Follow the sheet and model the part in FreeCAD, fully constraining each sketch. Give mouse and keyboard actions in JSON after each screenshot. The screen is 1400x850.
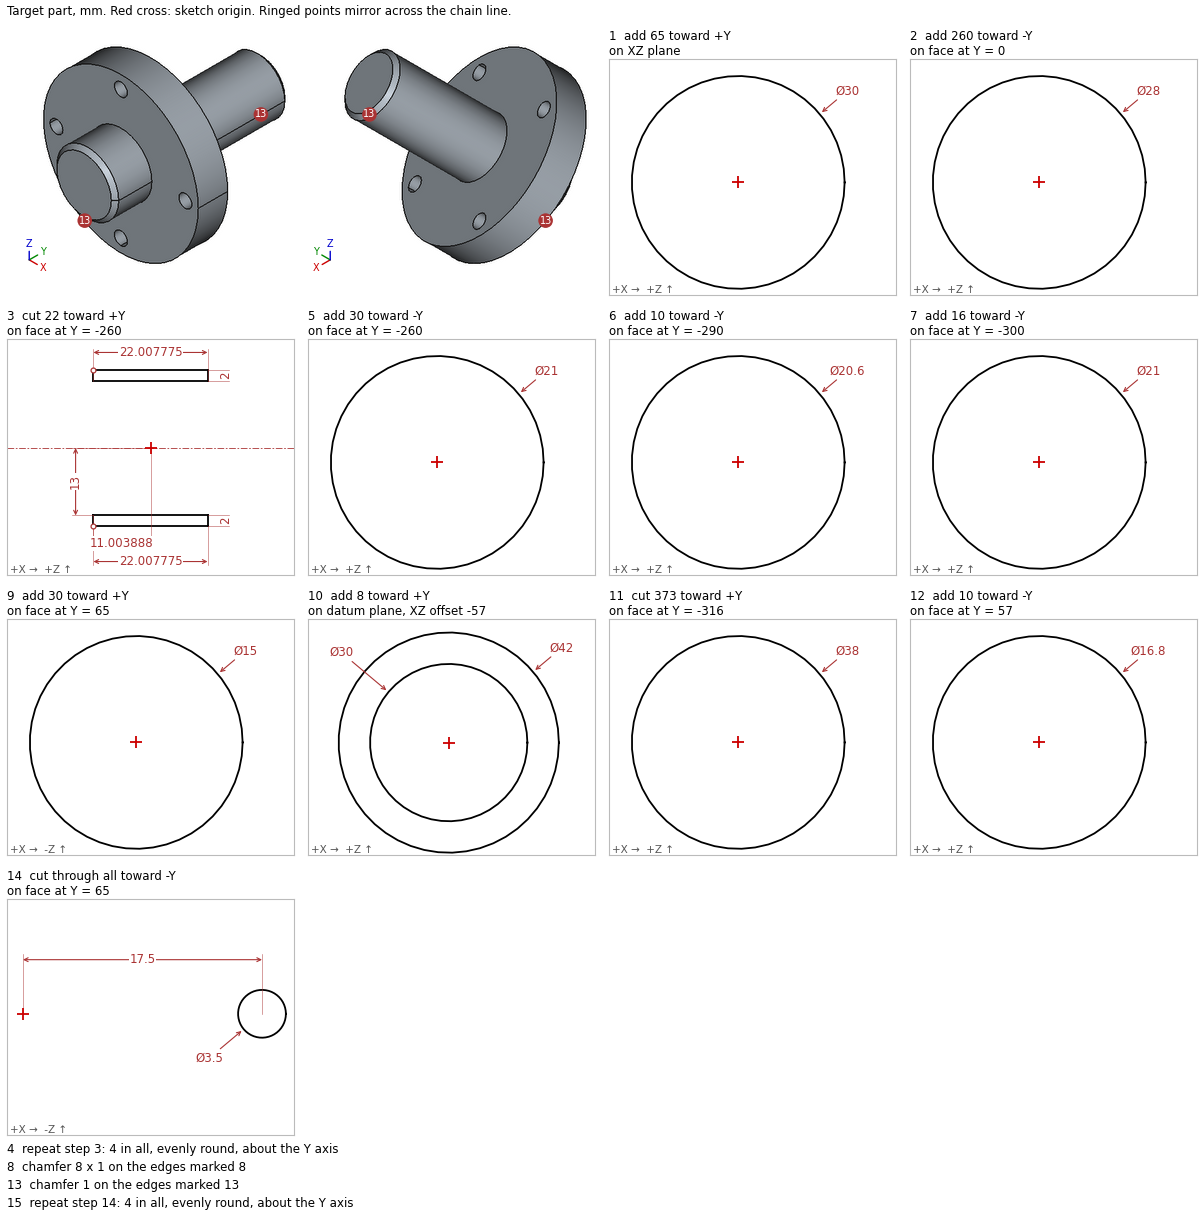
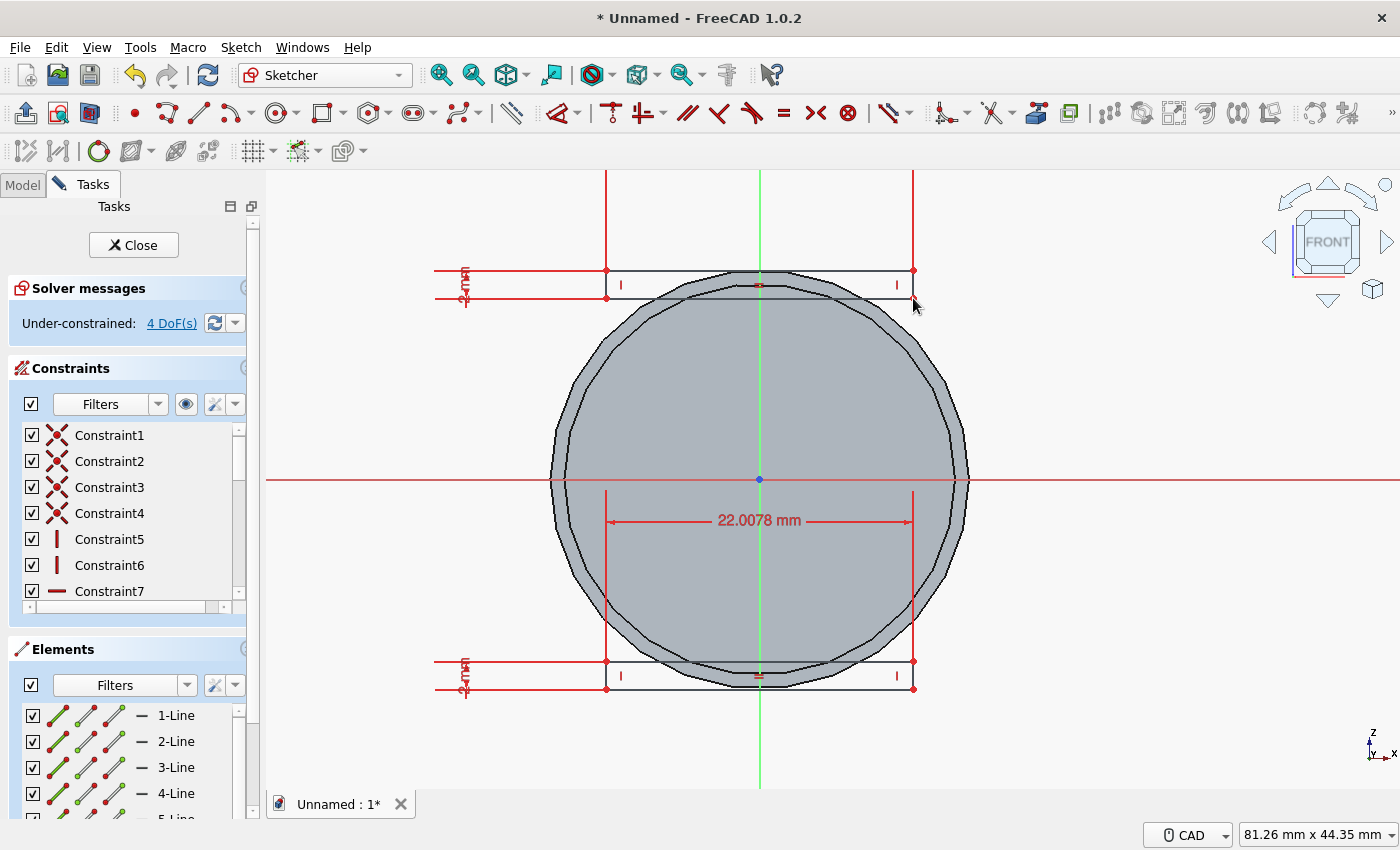
{"action": "left_click", "coordinate": [606, 690]}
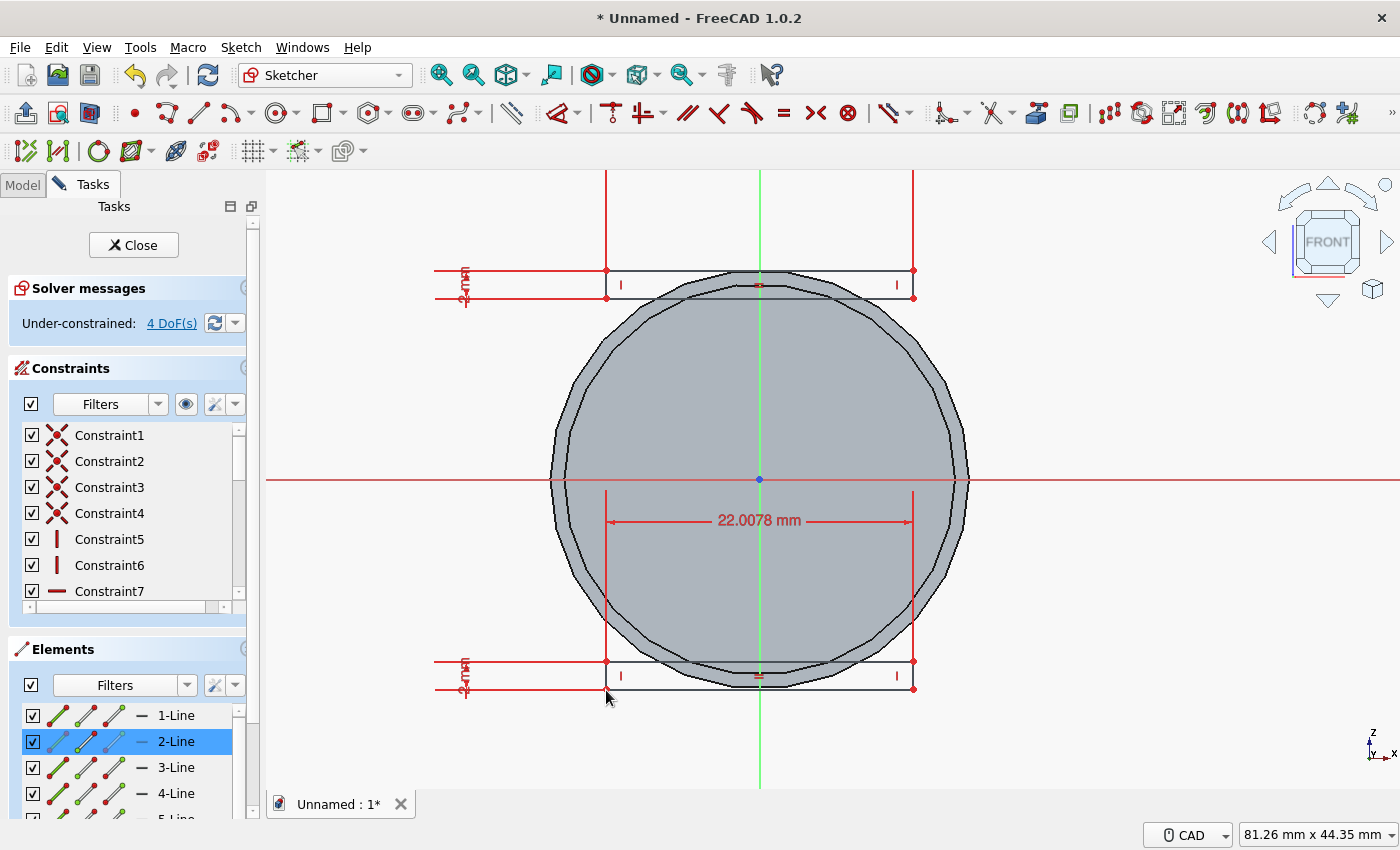
{"action": "left_click", "coordinate": [606, 271]}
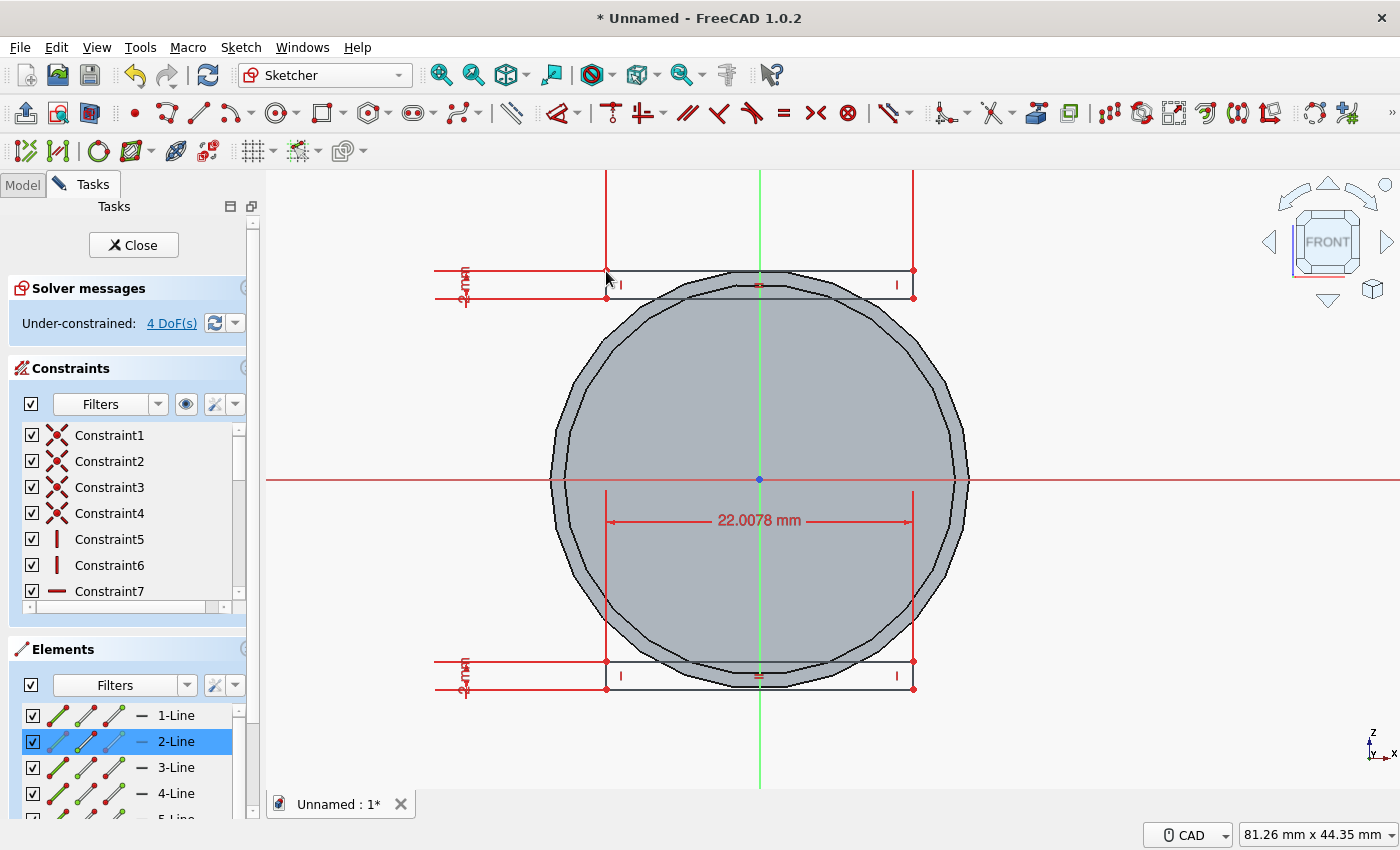
{"action": "left_click", "coordinate": [361, 480]}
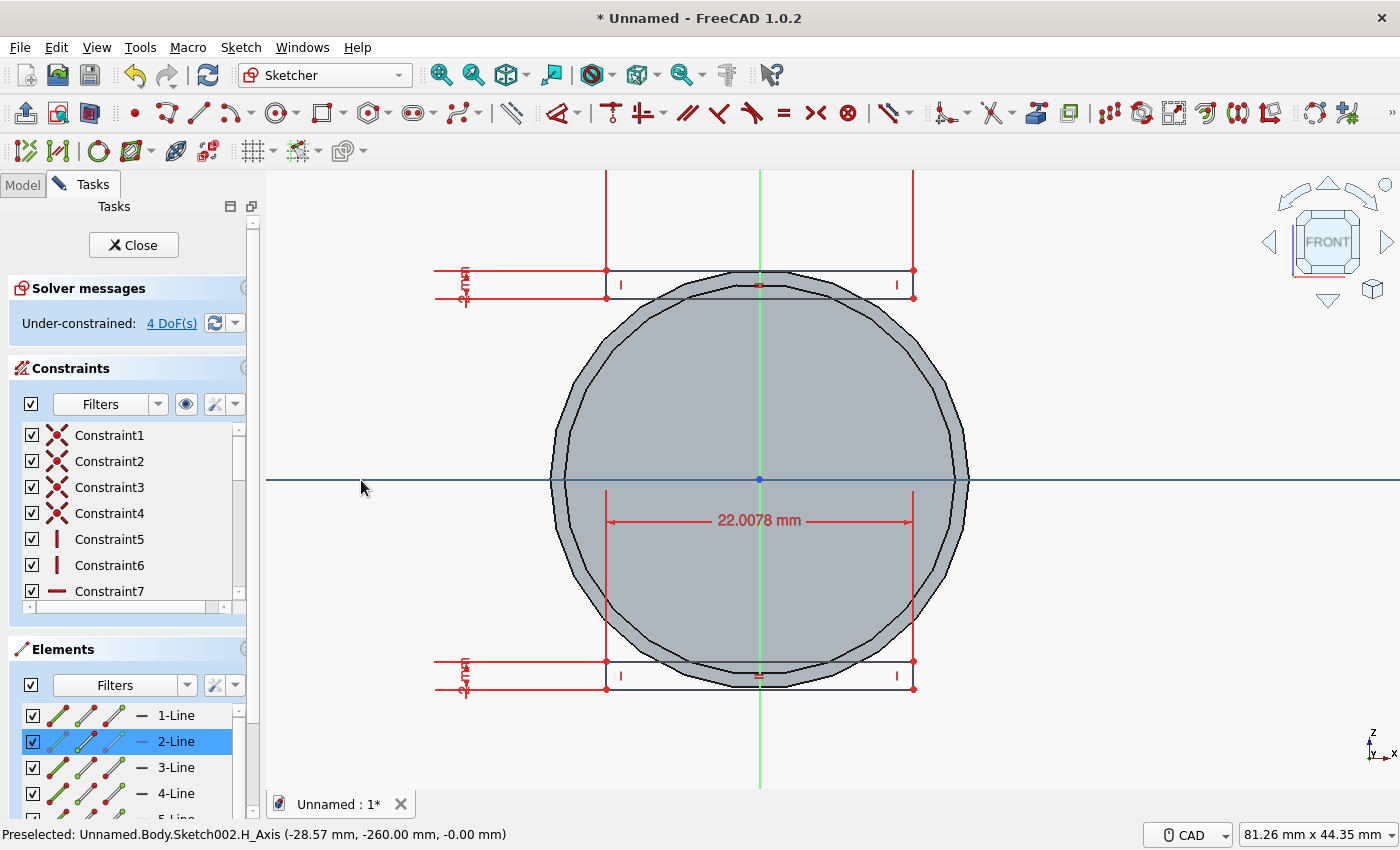
{"action": "left_click", "coordinate": [816, 114]}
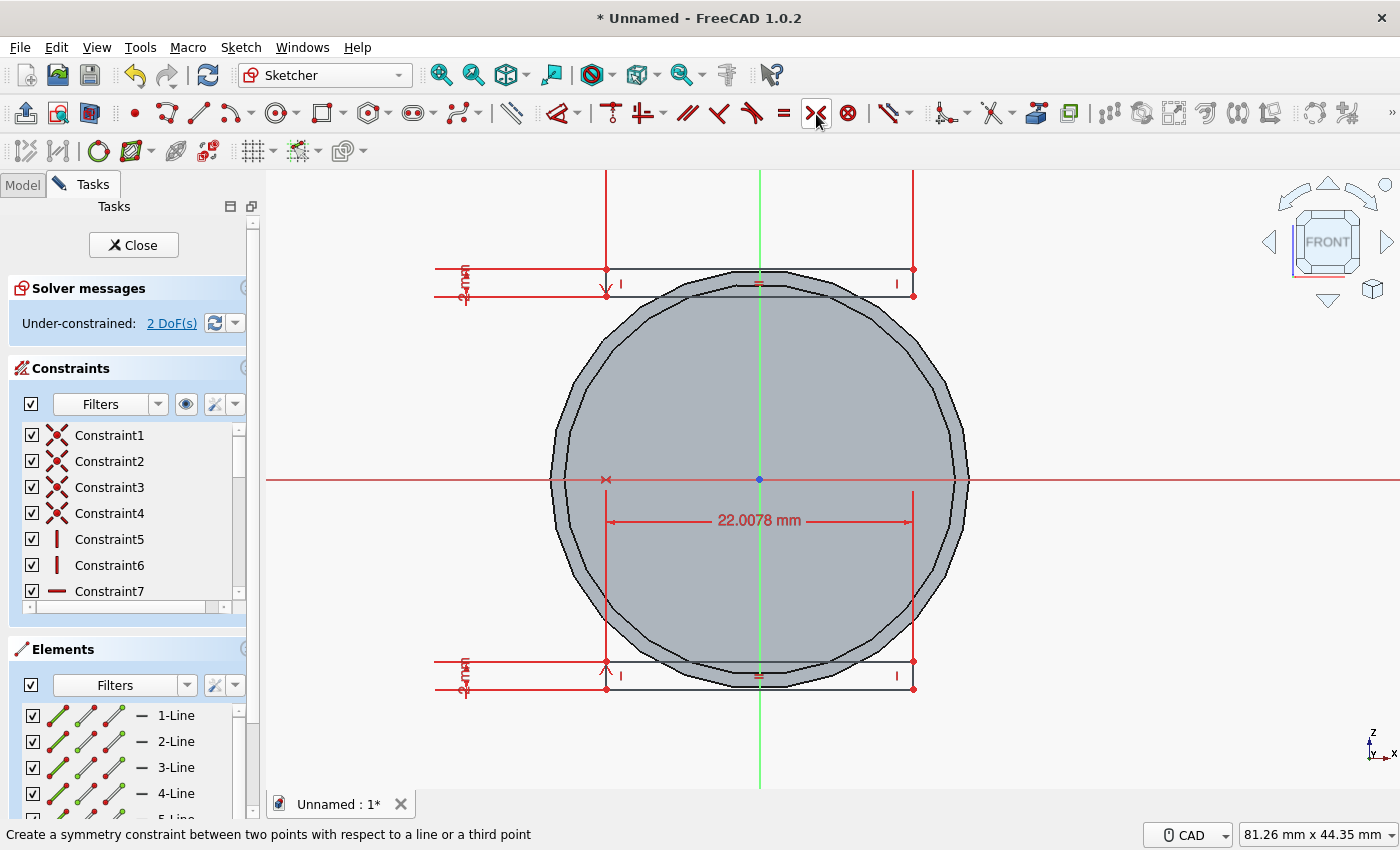
{"action": "left_click", "coordinate": [558, 114]}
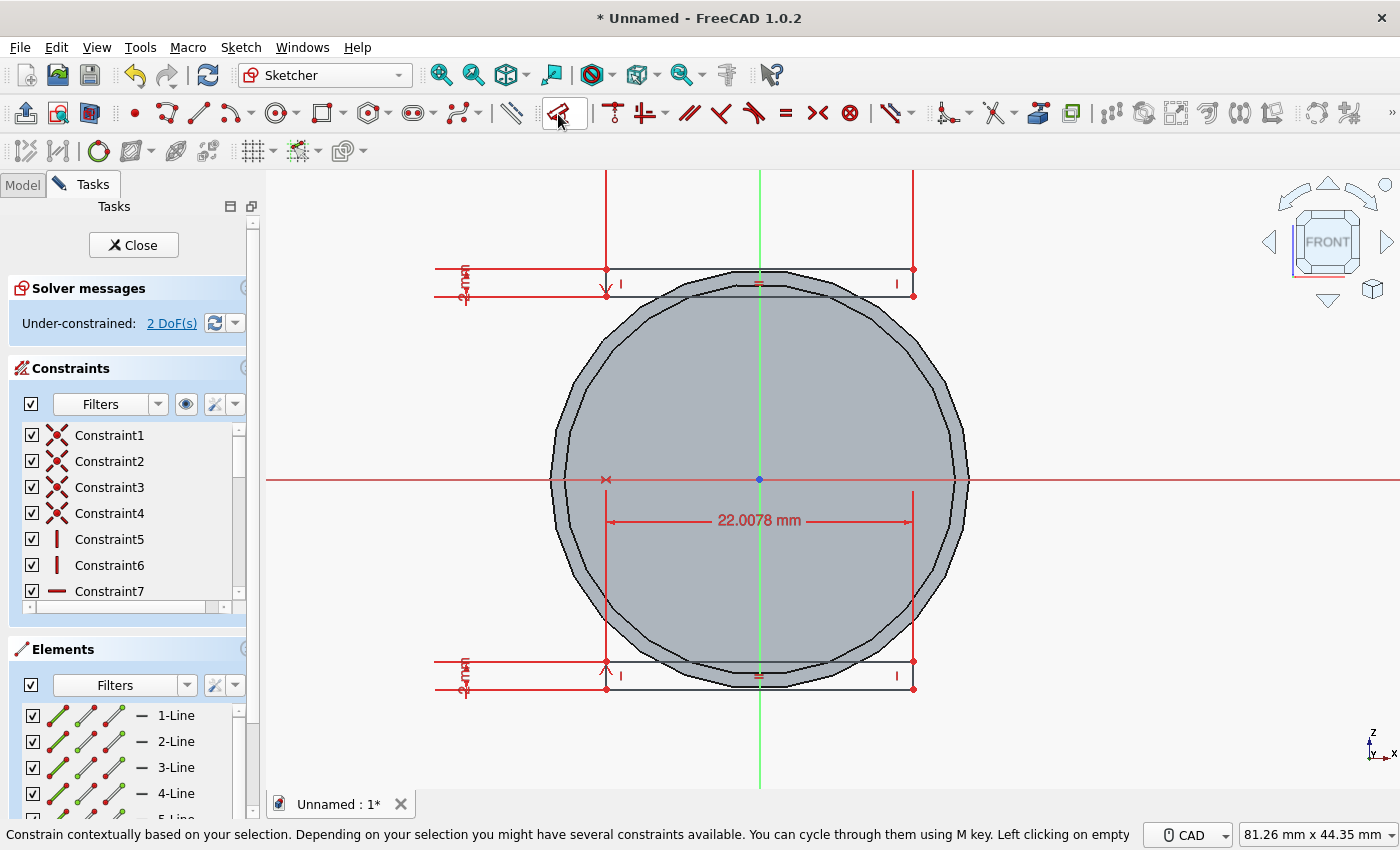
{"action": "left_click", "coordinate": [606, 662]}
{"action": "left_click", "coordinate": [572, 571]}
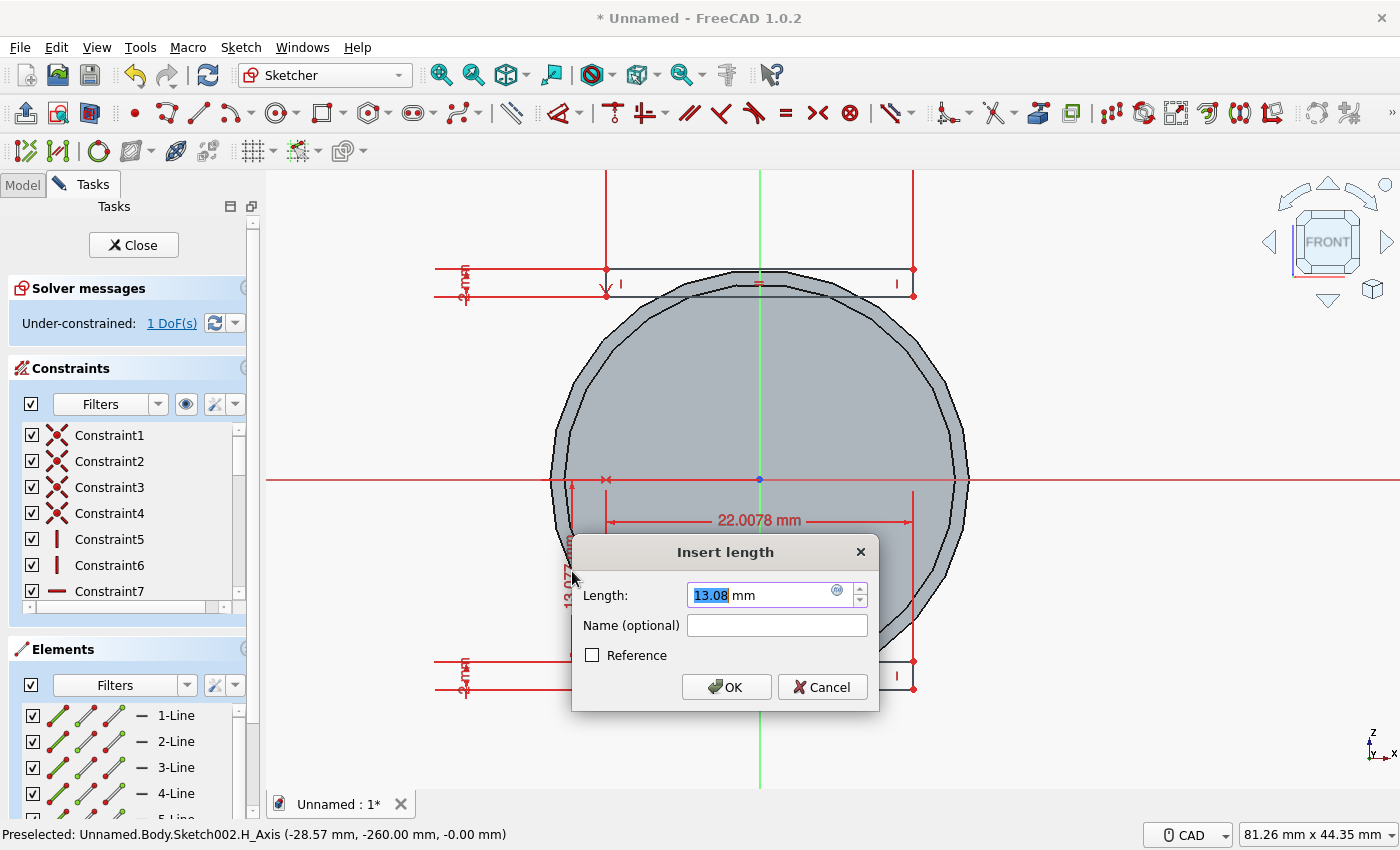
{"action": "type", "text": "13"}
{"action": "key", "text": "Return"}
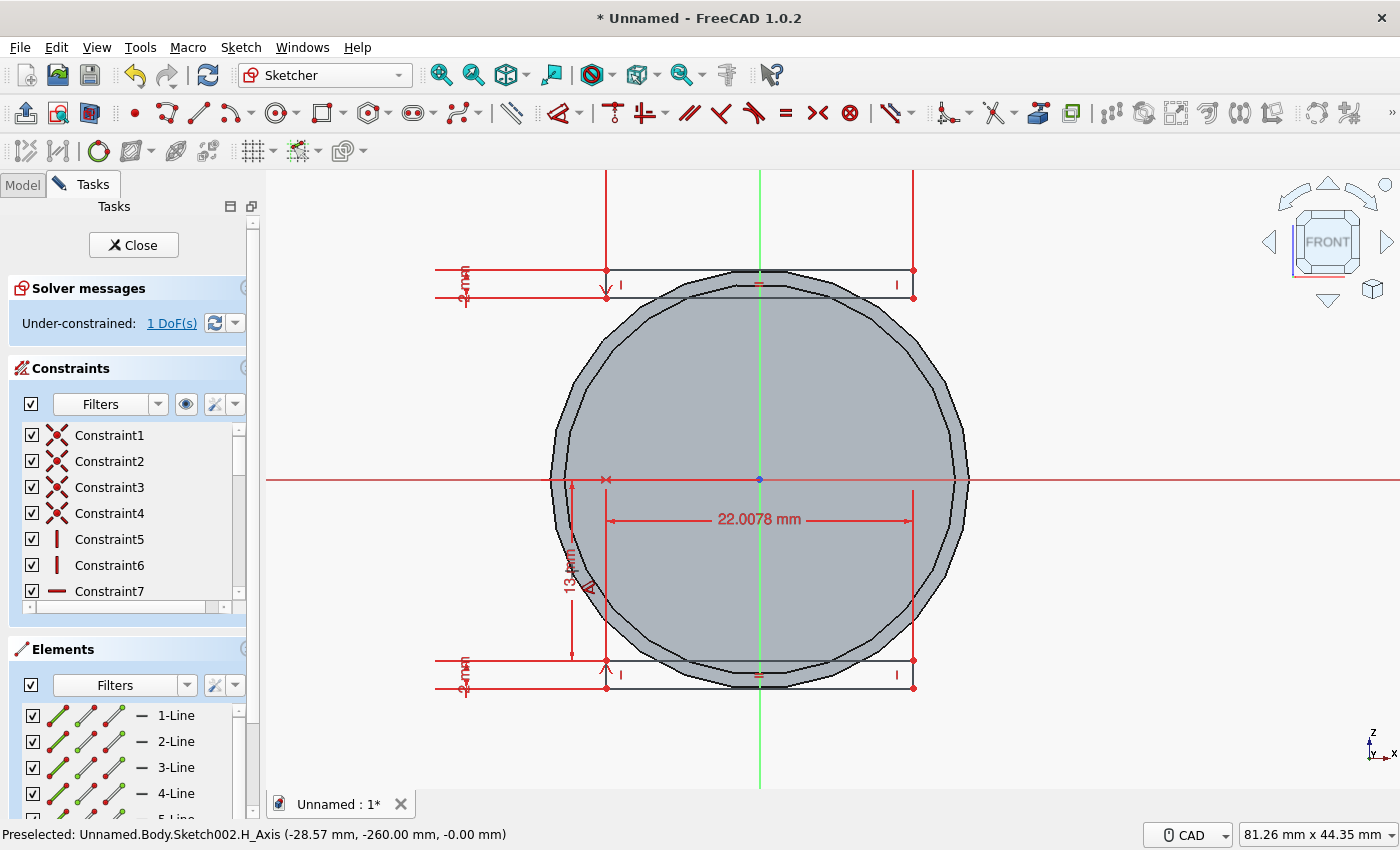
{"action": "left_click", "coordinate": [606, 661]}
{"action": "left_click", "coordinate": [683, 446]}